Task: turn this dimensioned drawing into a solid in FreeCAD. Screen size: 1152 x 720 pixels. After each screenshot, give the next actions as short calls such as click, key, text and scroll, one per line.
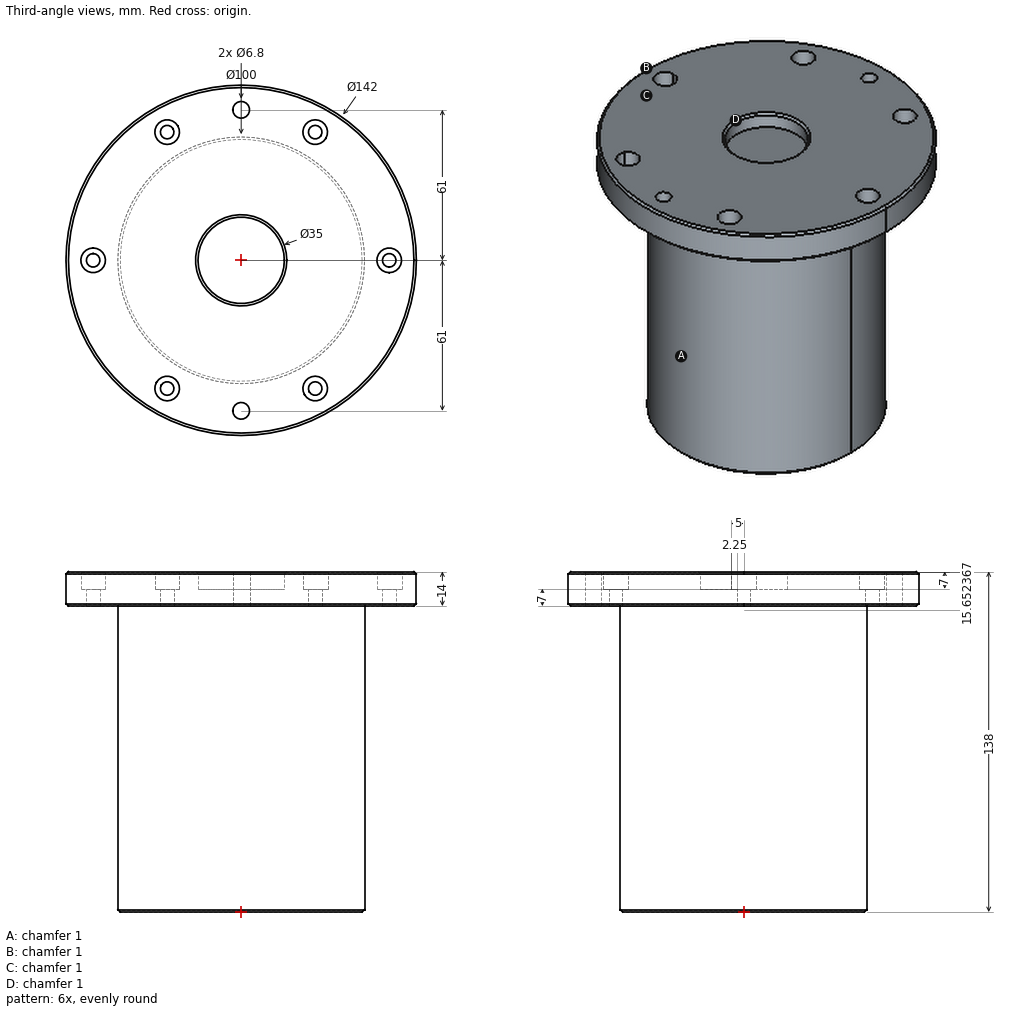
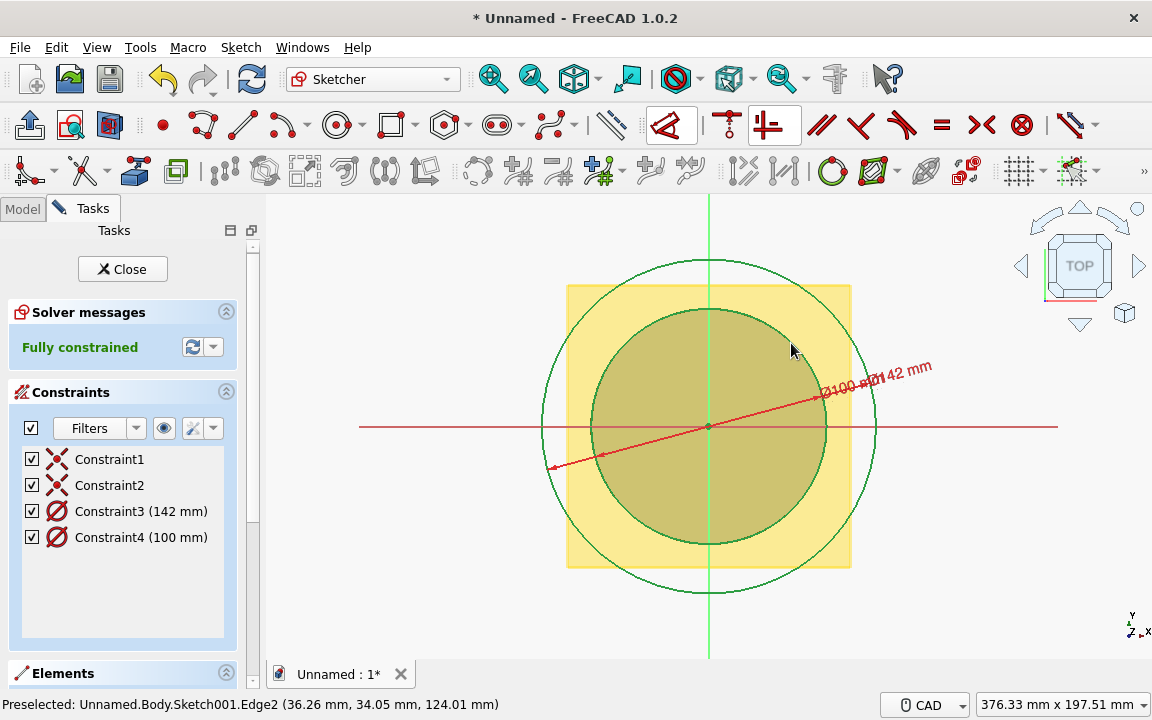
click(123, 269)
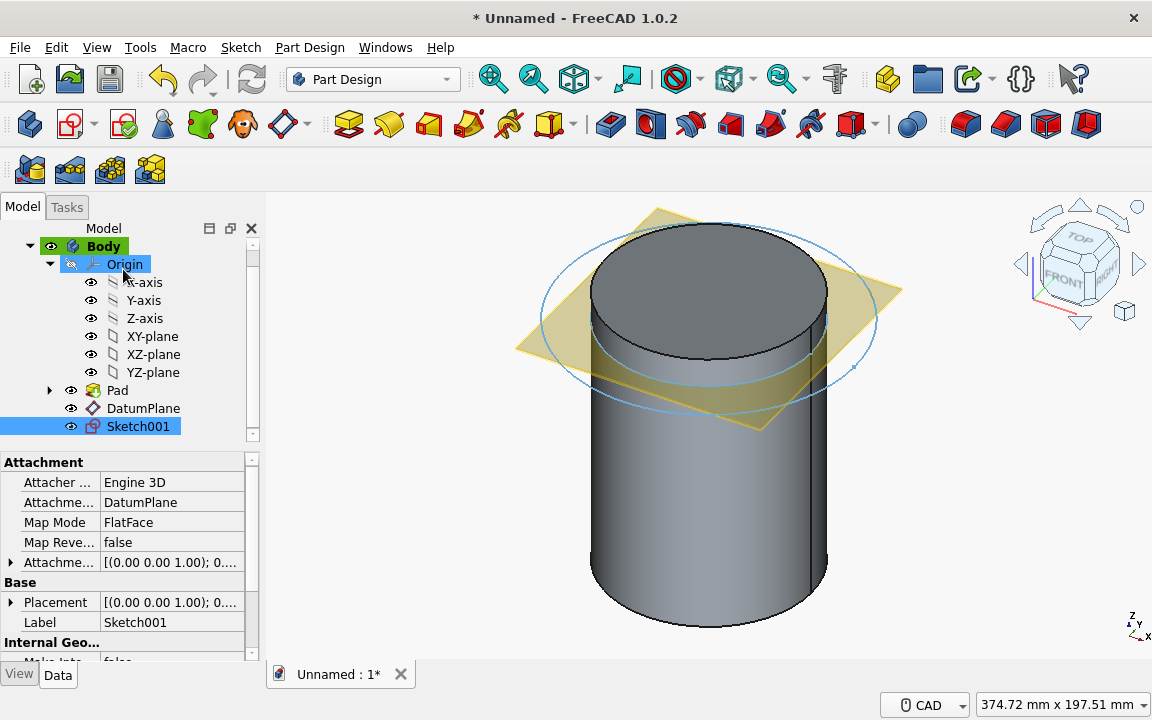
click(350, 124)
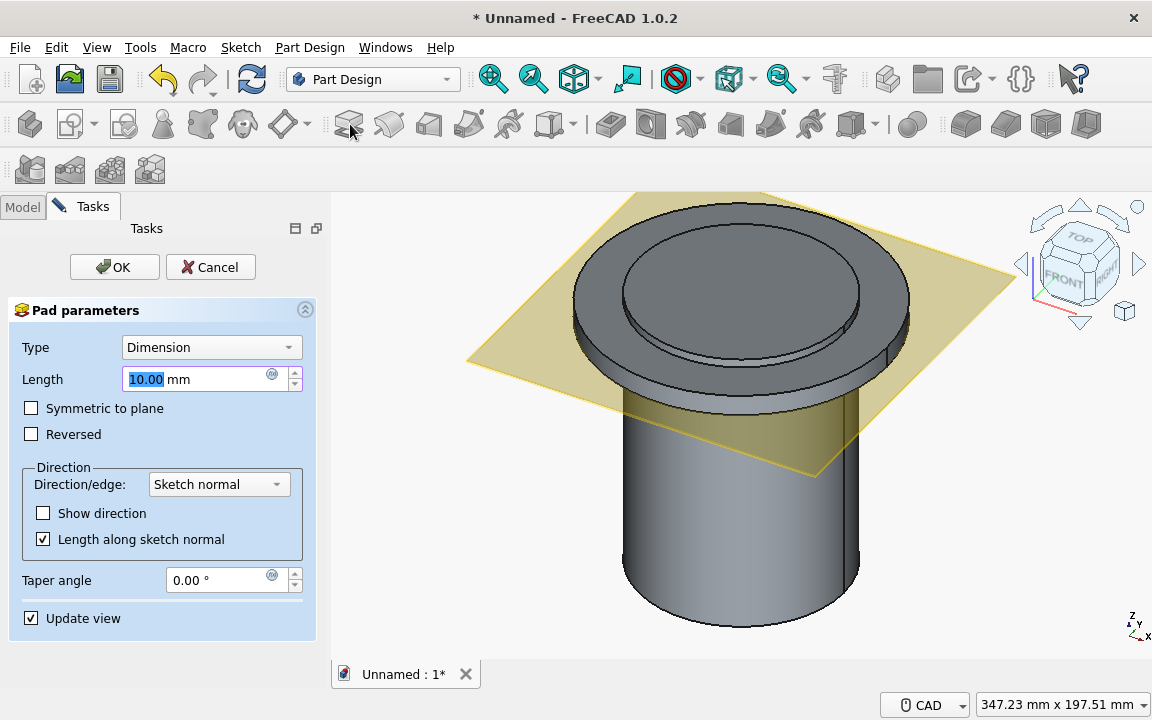
text(14)
key(Tab)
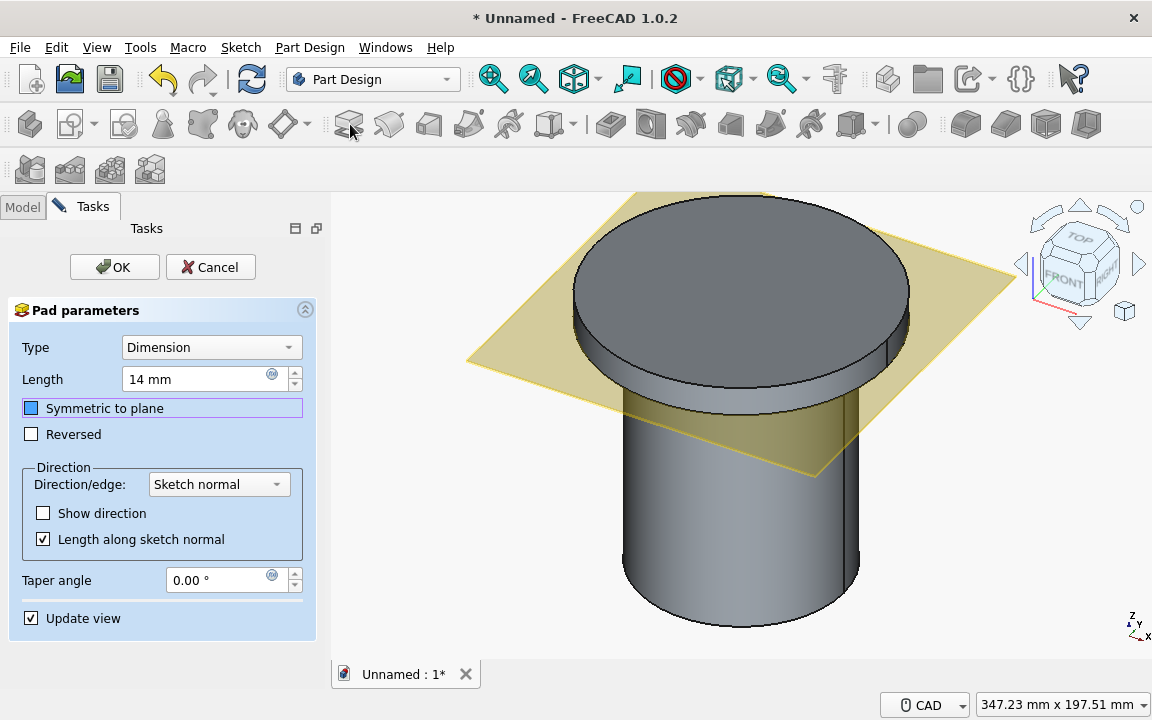
click(115, 267)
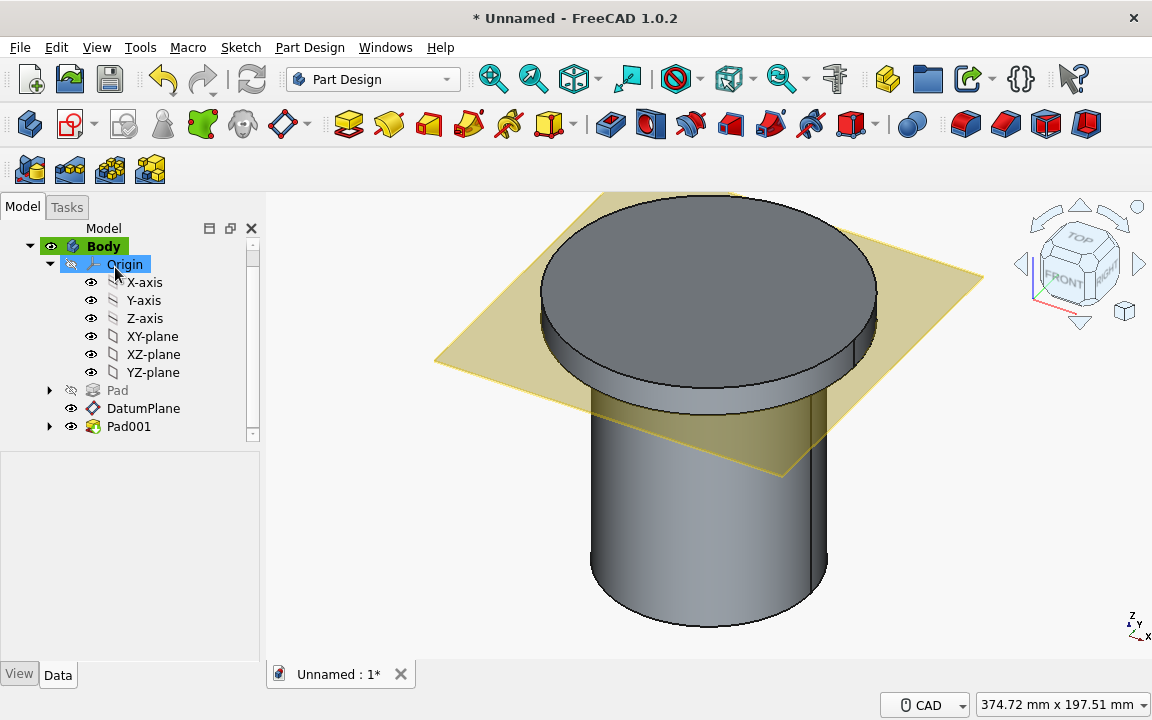
click(116, 408)
key(space)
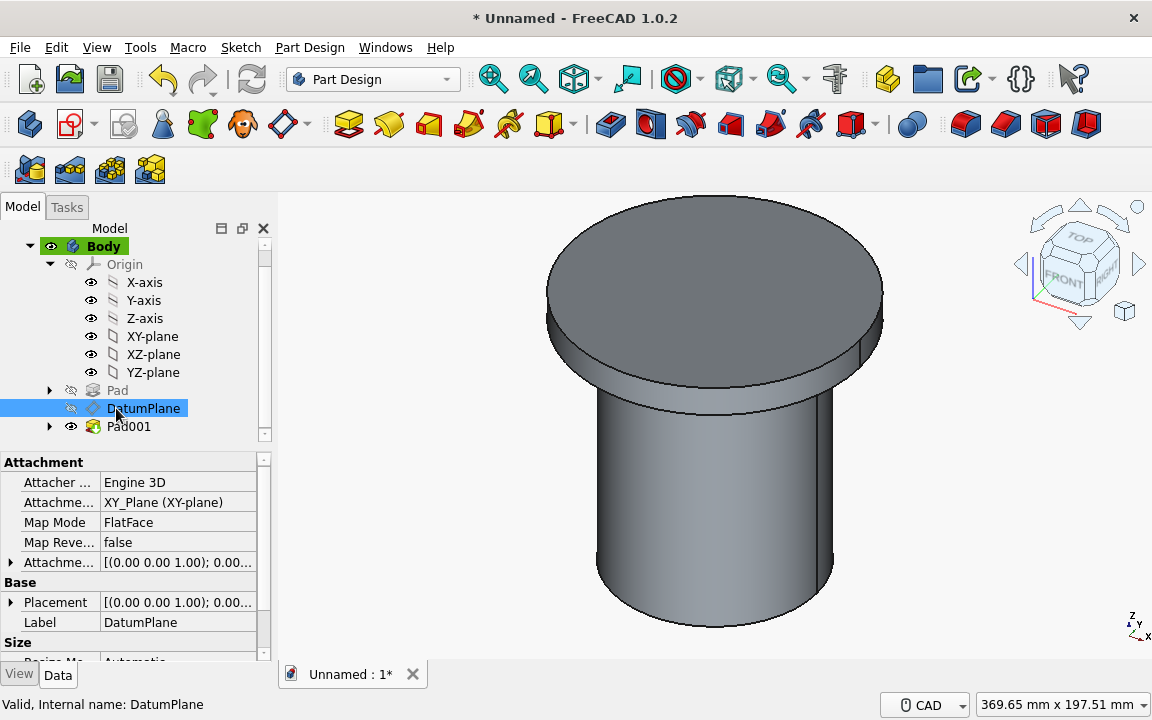
key(v)
key(f)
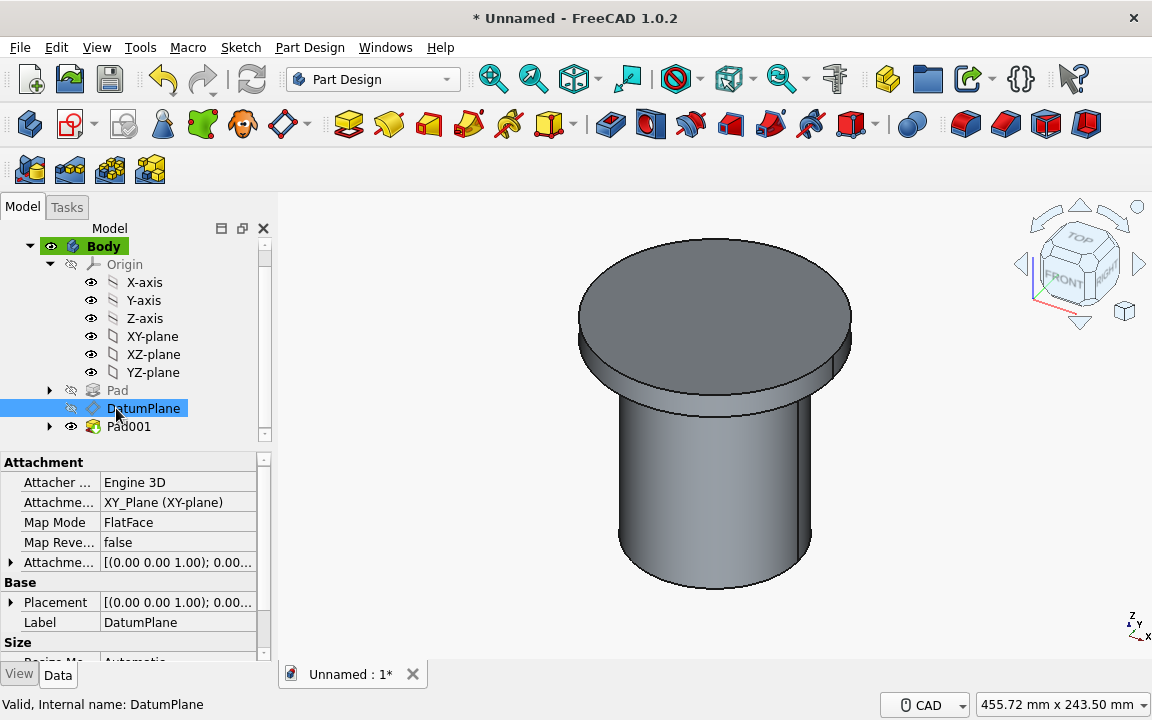
click(806, 551)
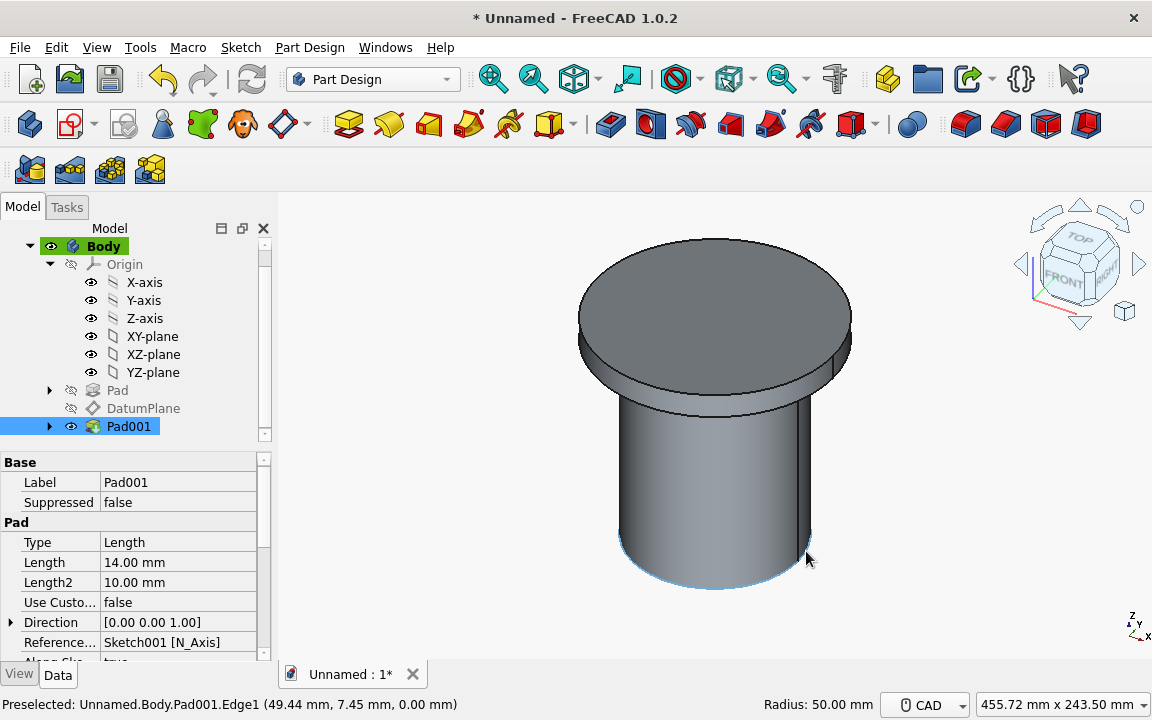
click(1006, 124)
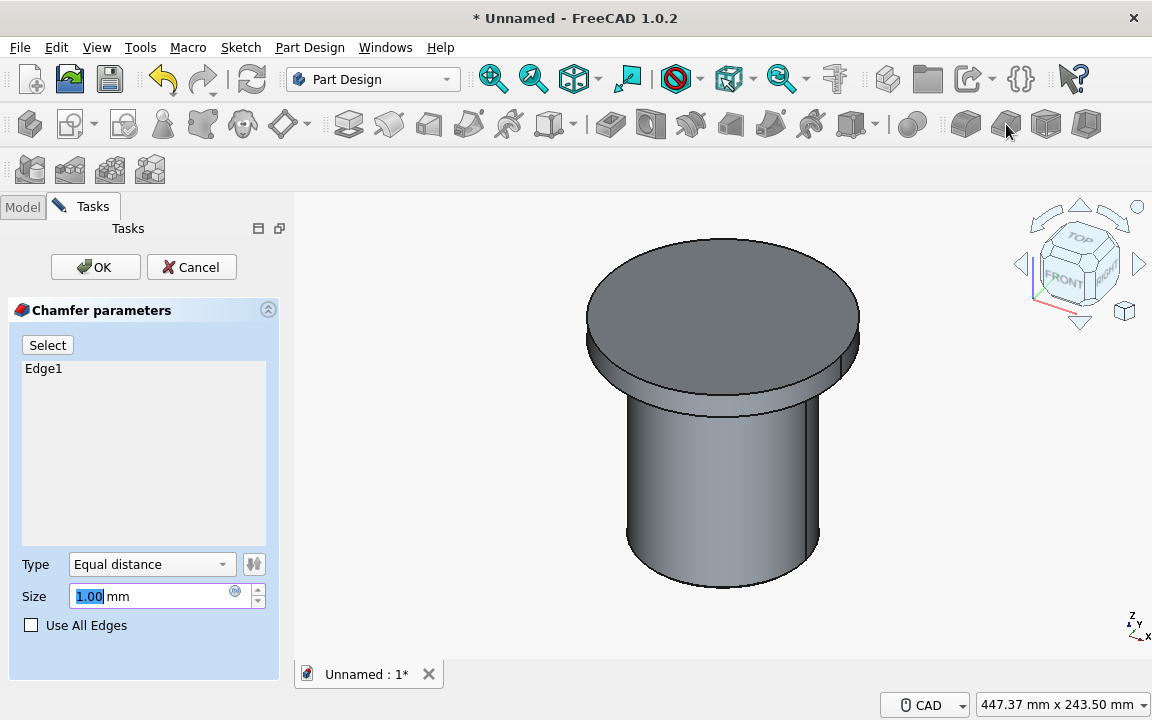
text(1)
key(Tab)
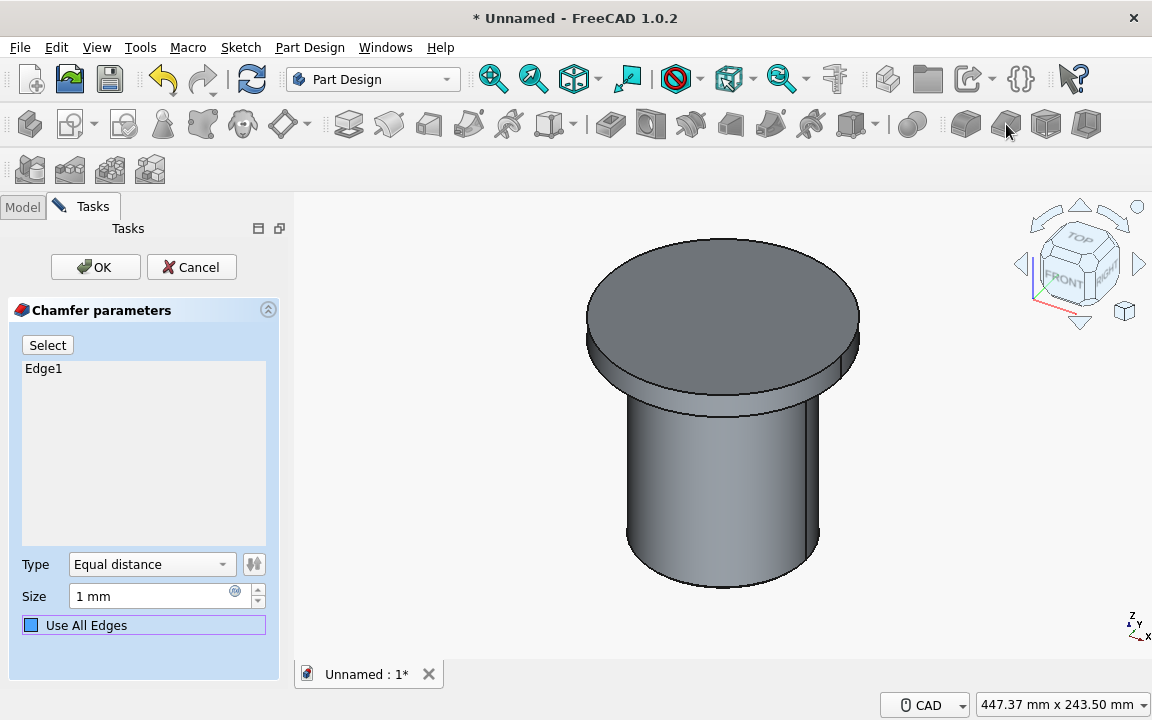
click(96, 267)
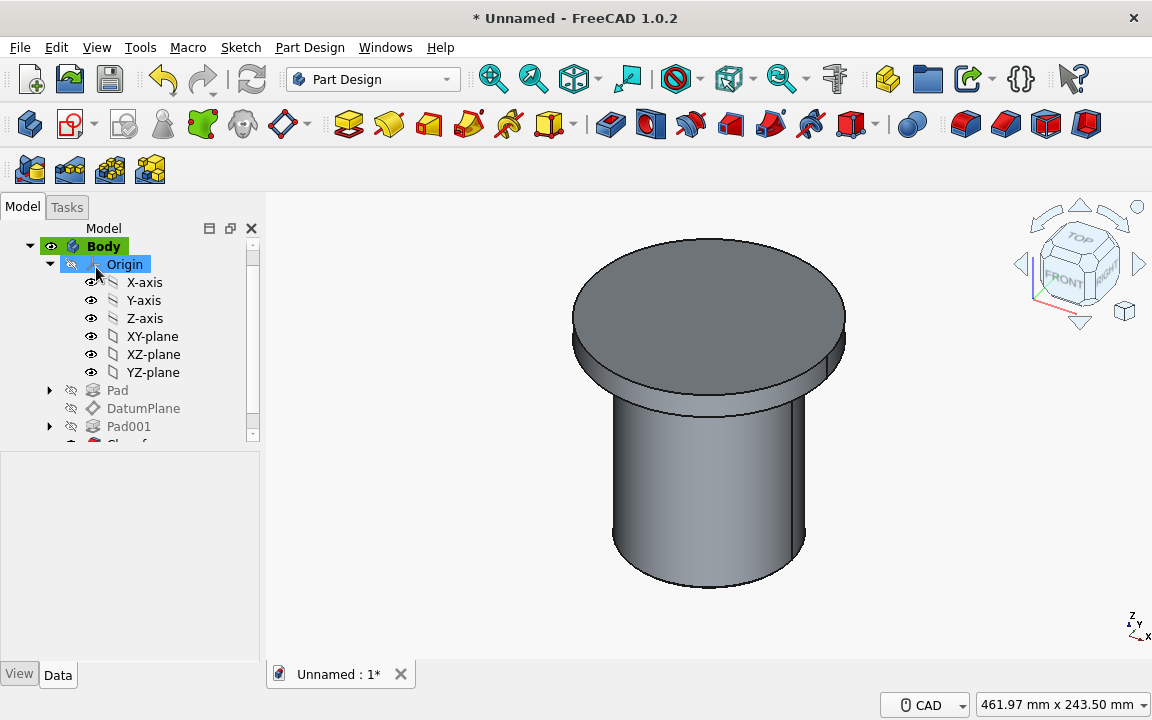
click(574, 324)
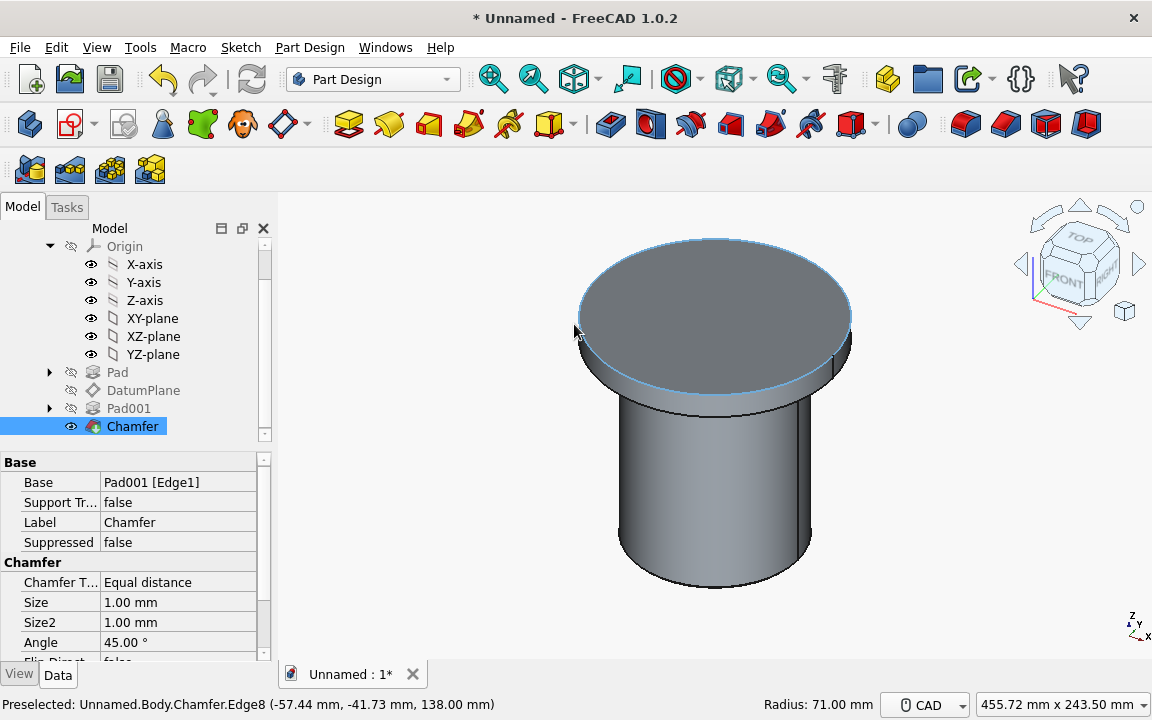
click(1006, 124)